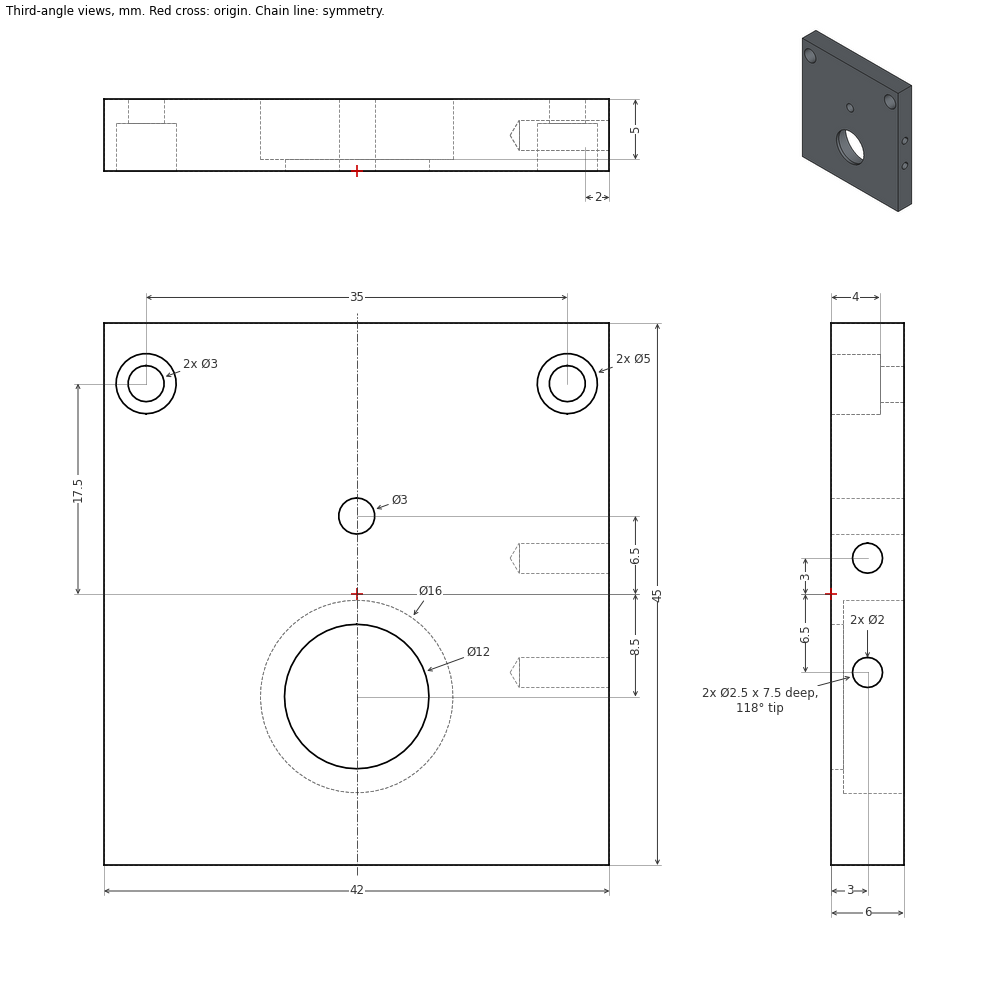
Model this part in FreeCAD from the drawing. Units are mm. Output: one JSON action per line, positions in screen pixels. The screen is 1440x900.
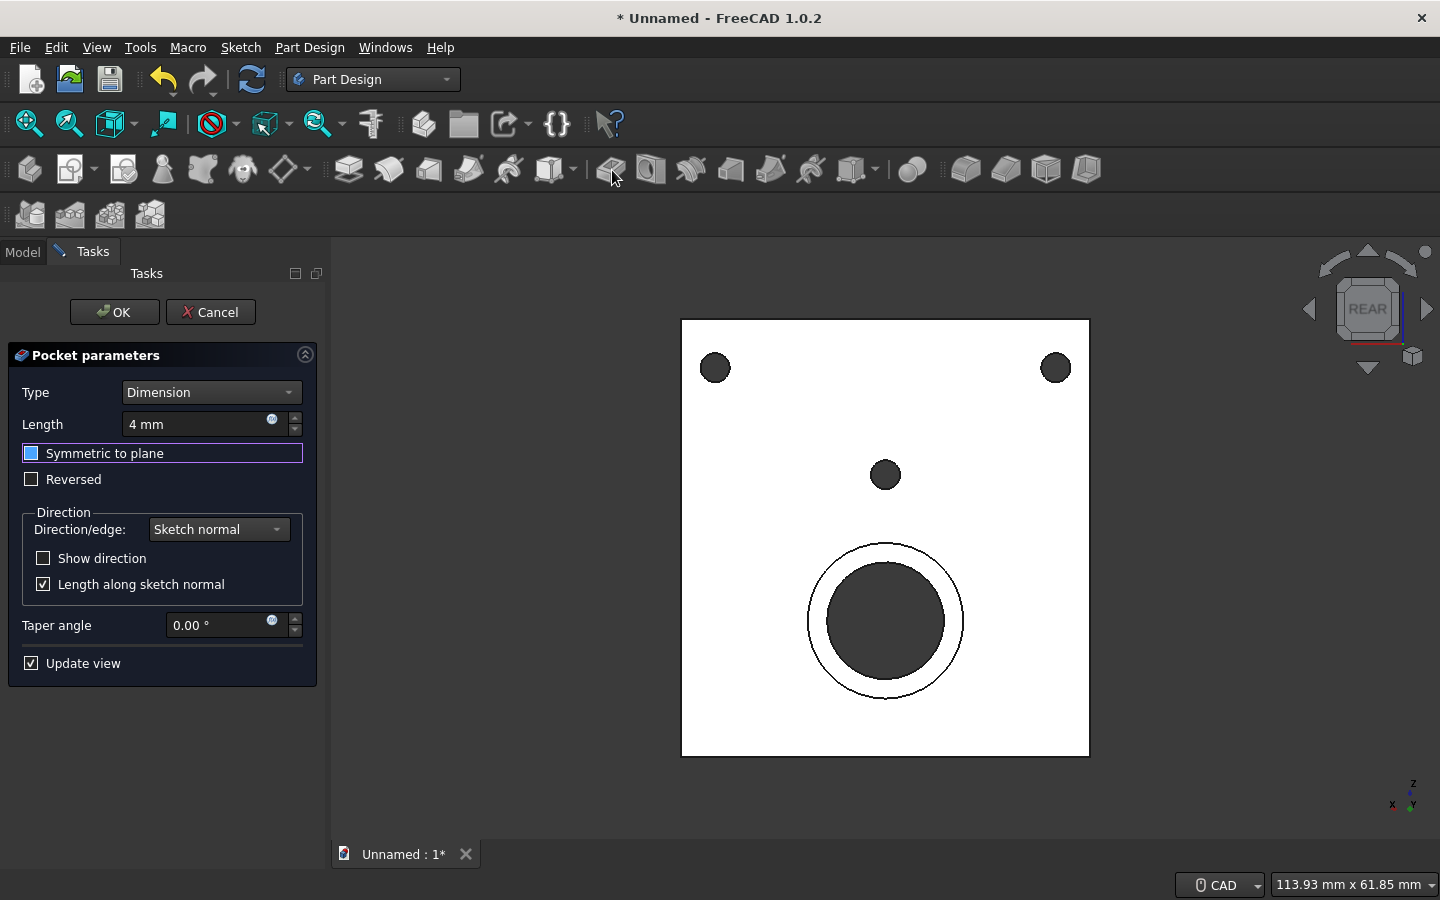
{"action": "left_click", "coordinate": [115, 312]}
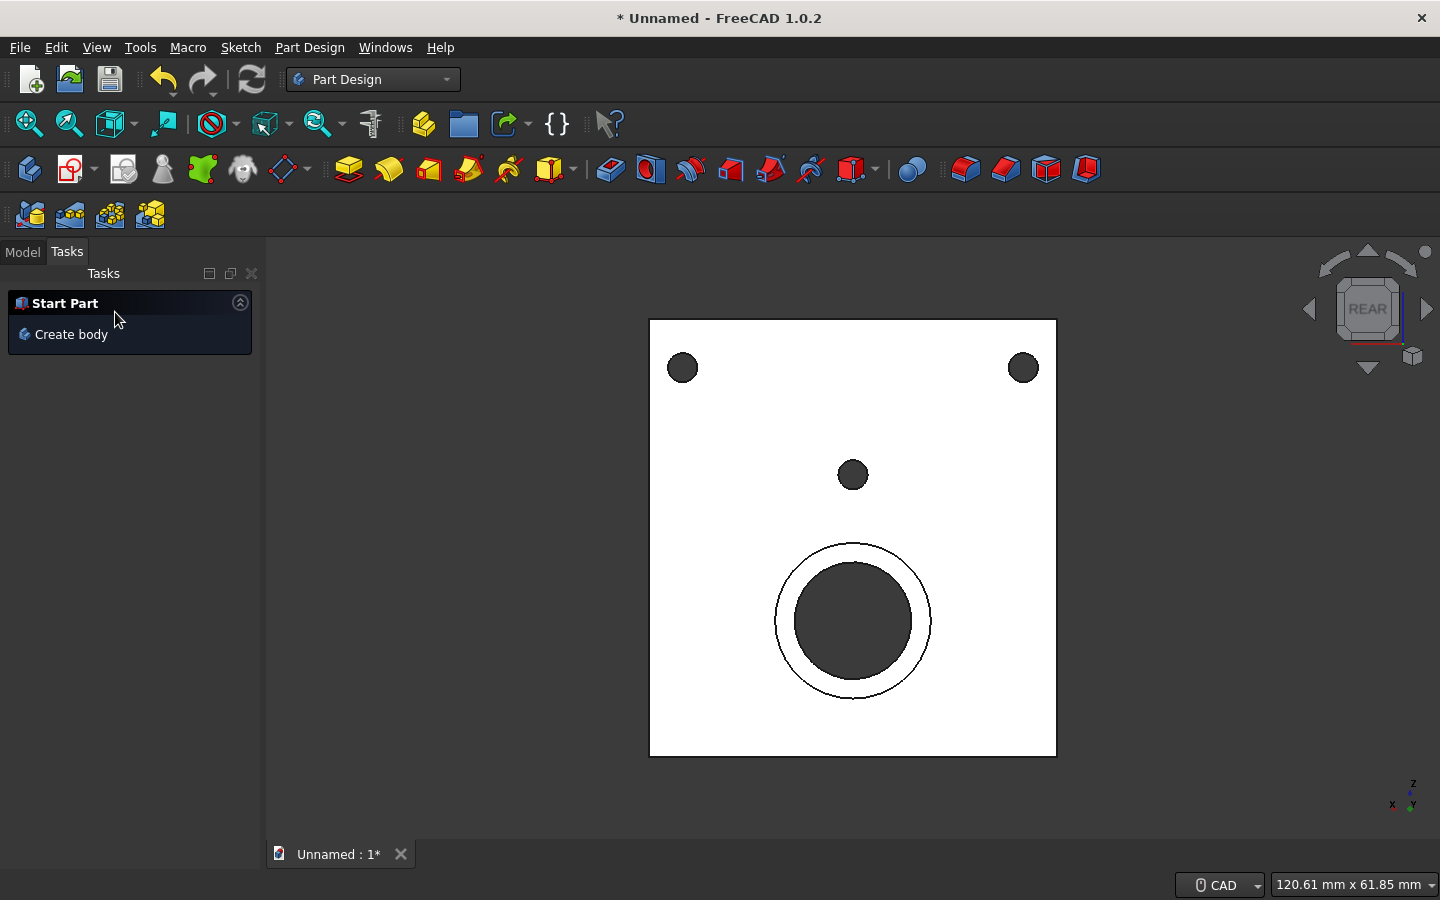
{"action": "key", "text": "0"}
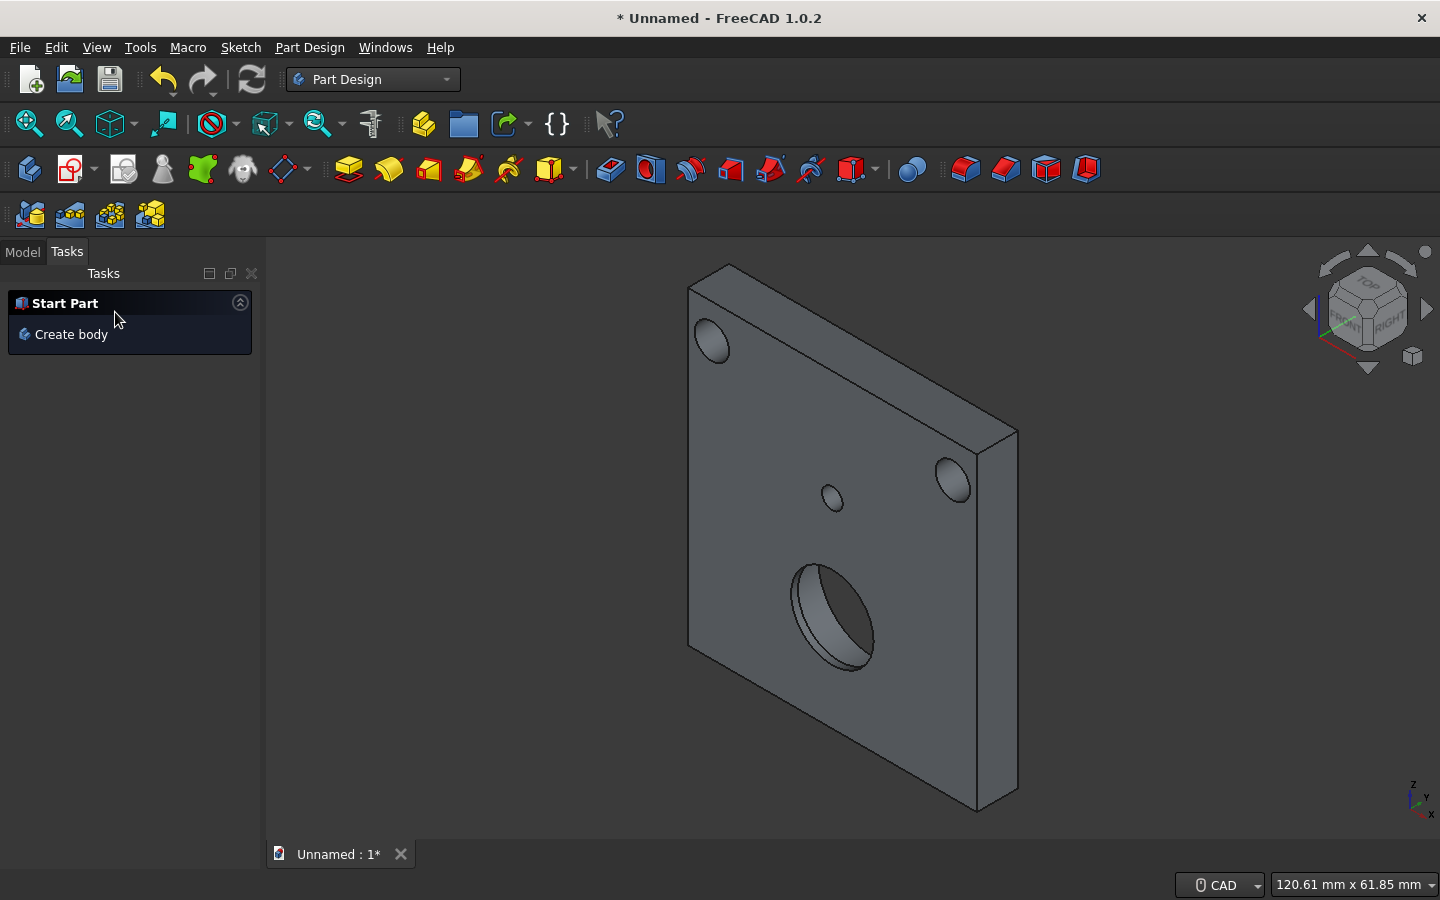
{"action": "left_click", "coordinate": [998, 518]}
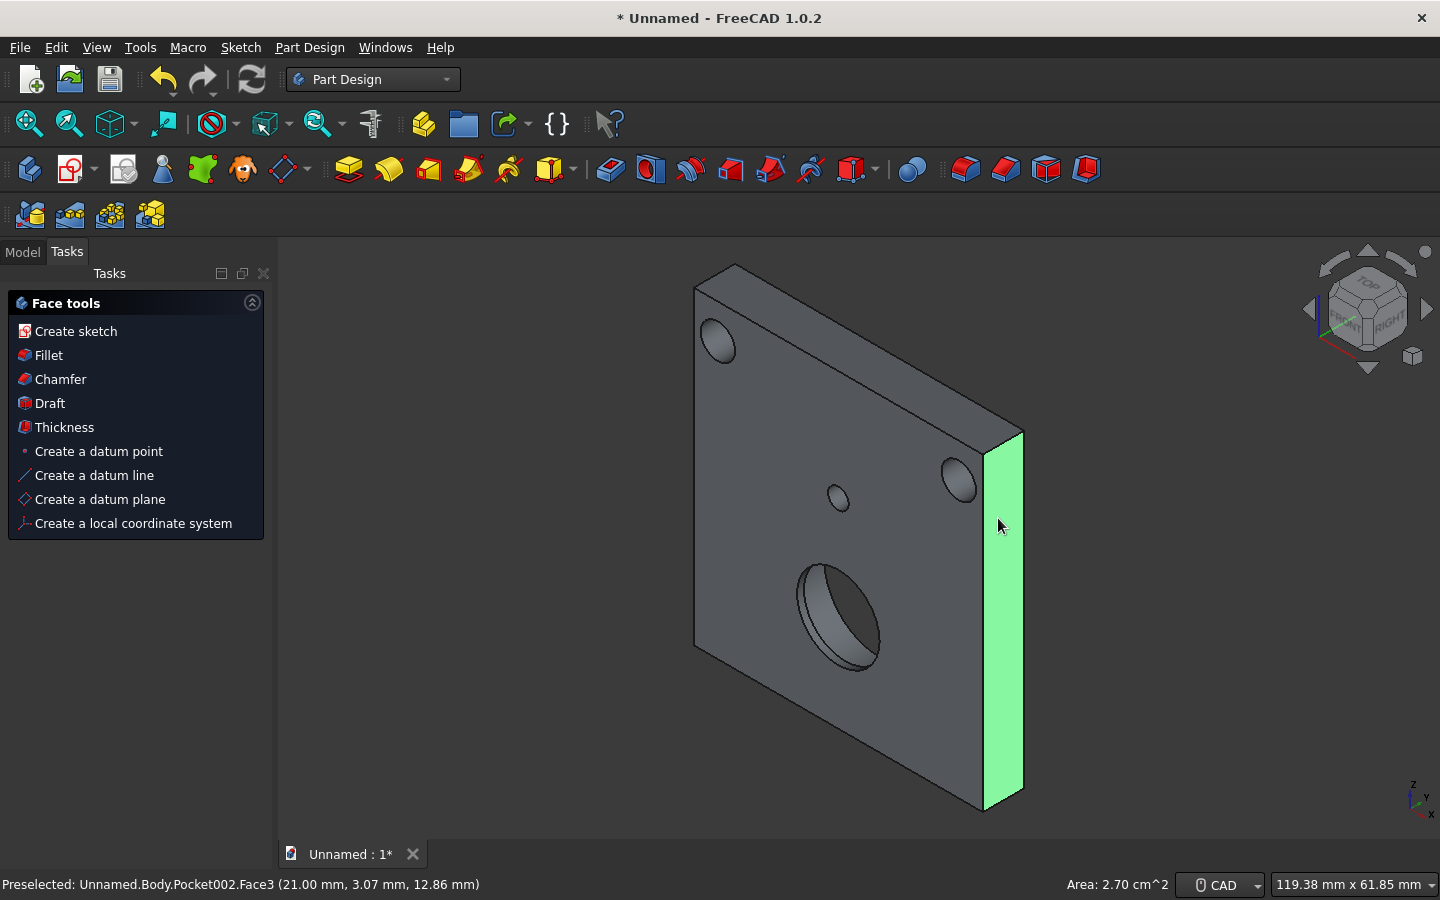
{"action": "left_click", "coordinate": [70, 170]}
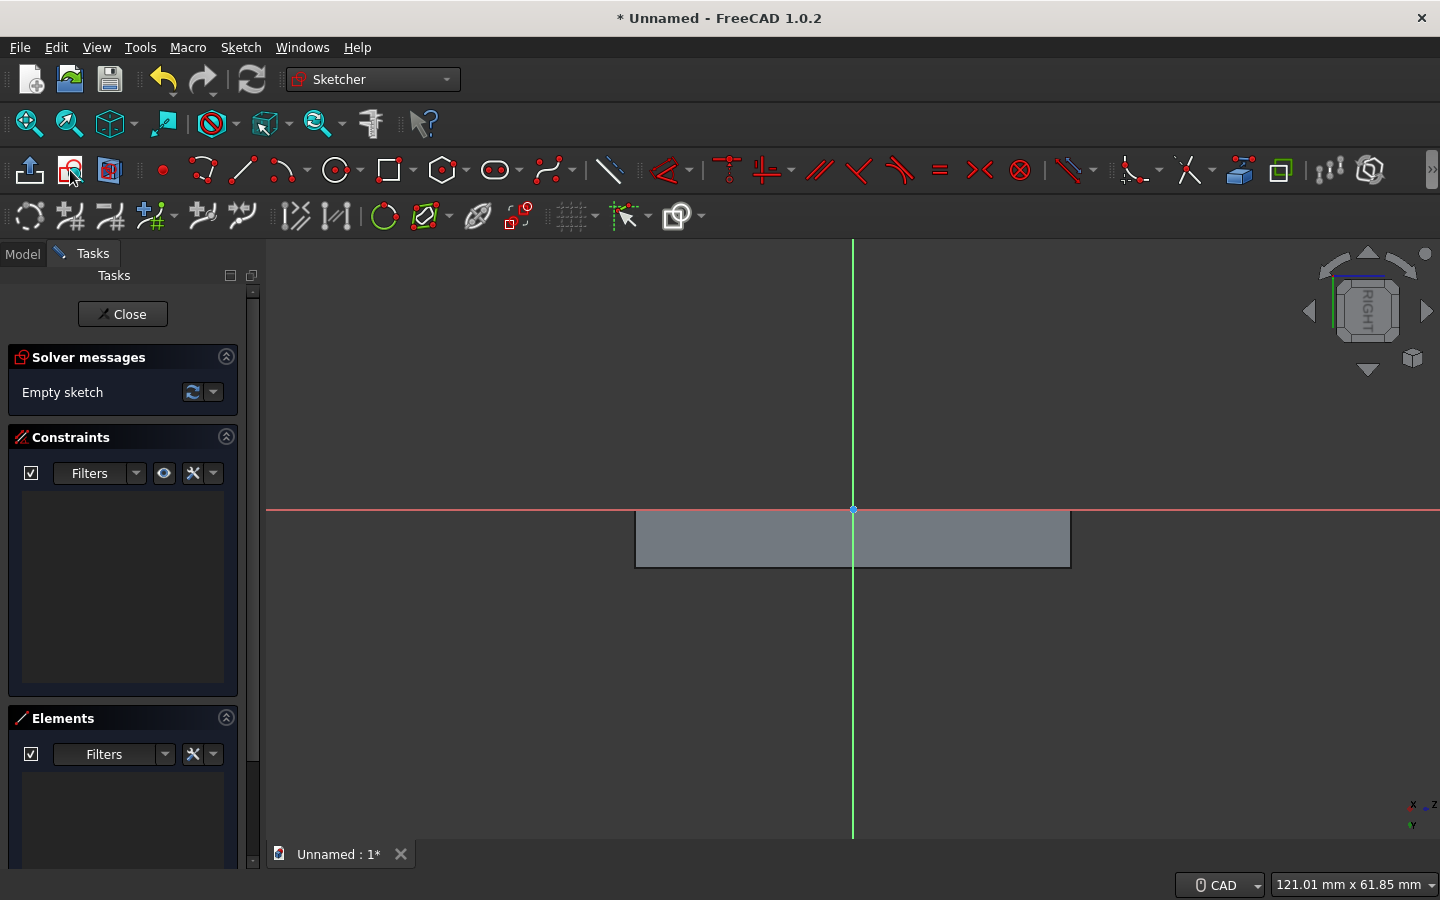
{"action": "scroll", "coordinate": [846, 527], "scroll_direction": "up", "scroll_amount": 9}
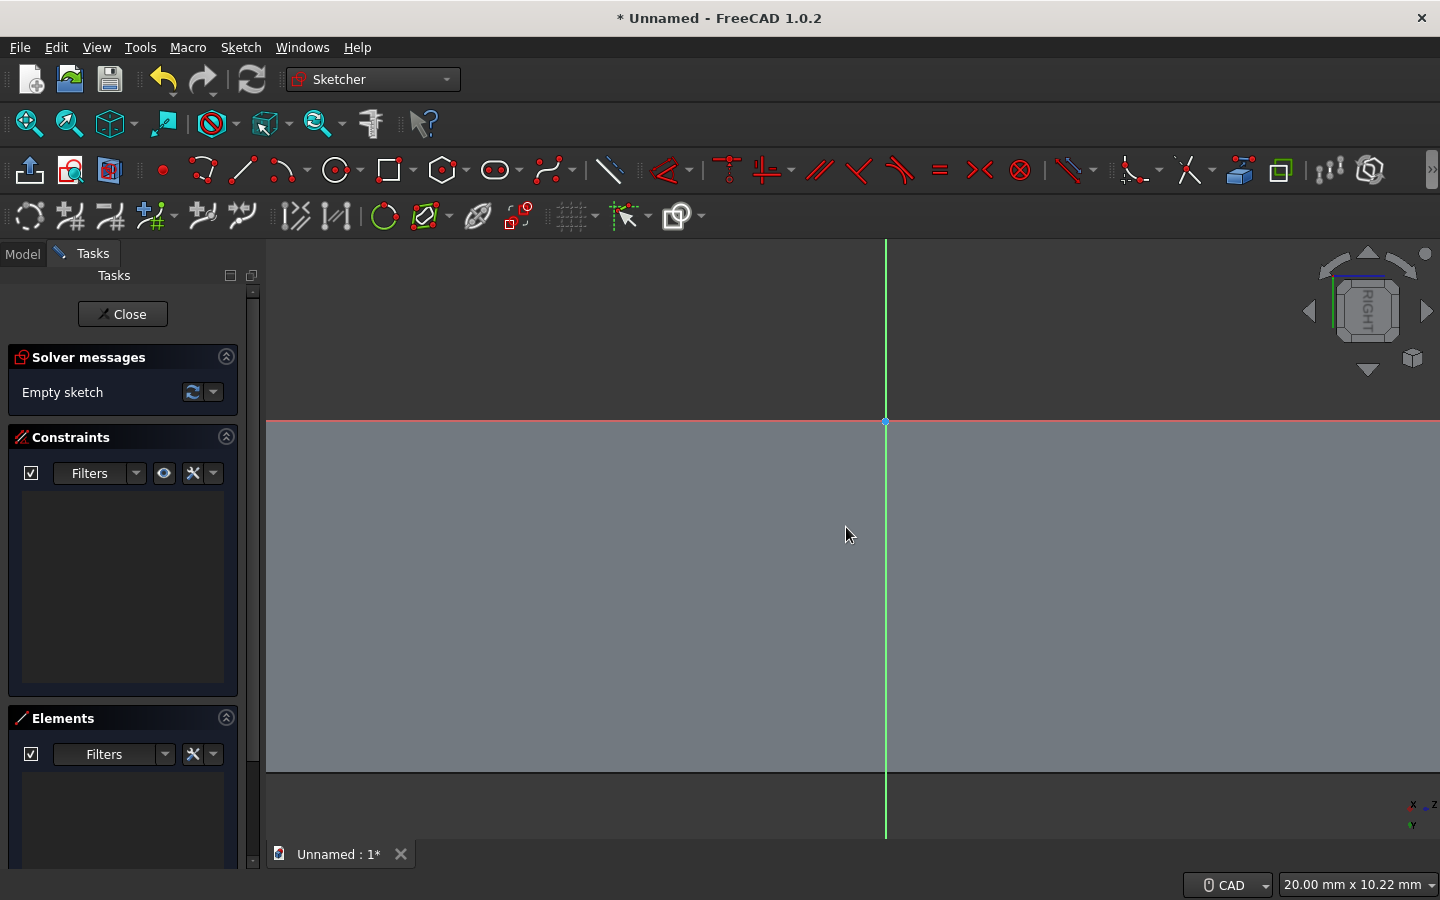
{"action": "key", "text": "g c"}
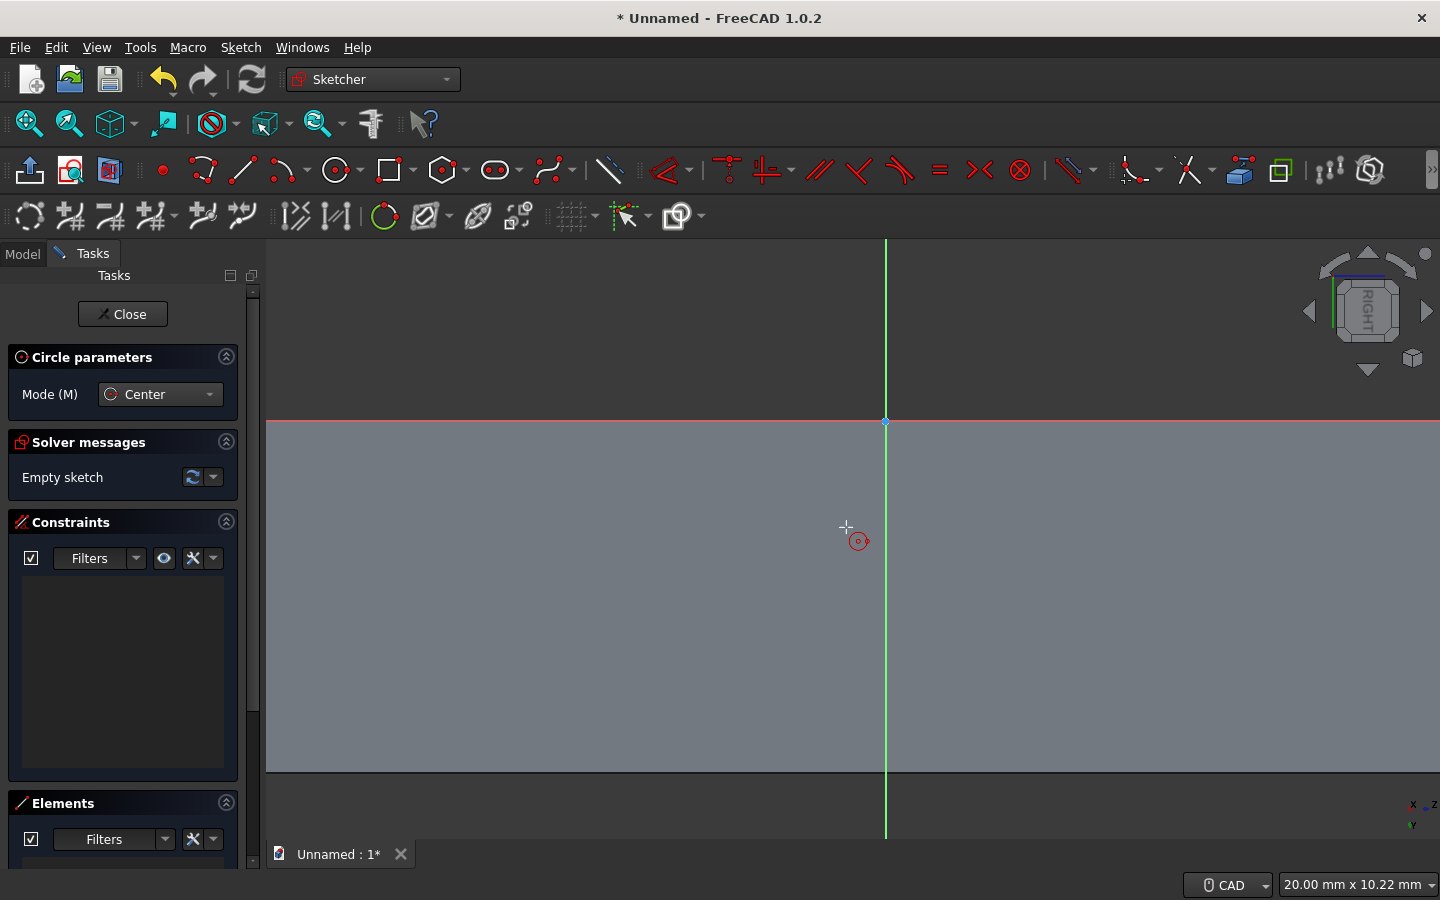
{"action": "left_click", "coordinate": [504, 597]}
{"action": "mouse_move", "coordinate": [546, 556]}